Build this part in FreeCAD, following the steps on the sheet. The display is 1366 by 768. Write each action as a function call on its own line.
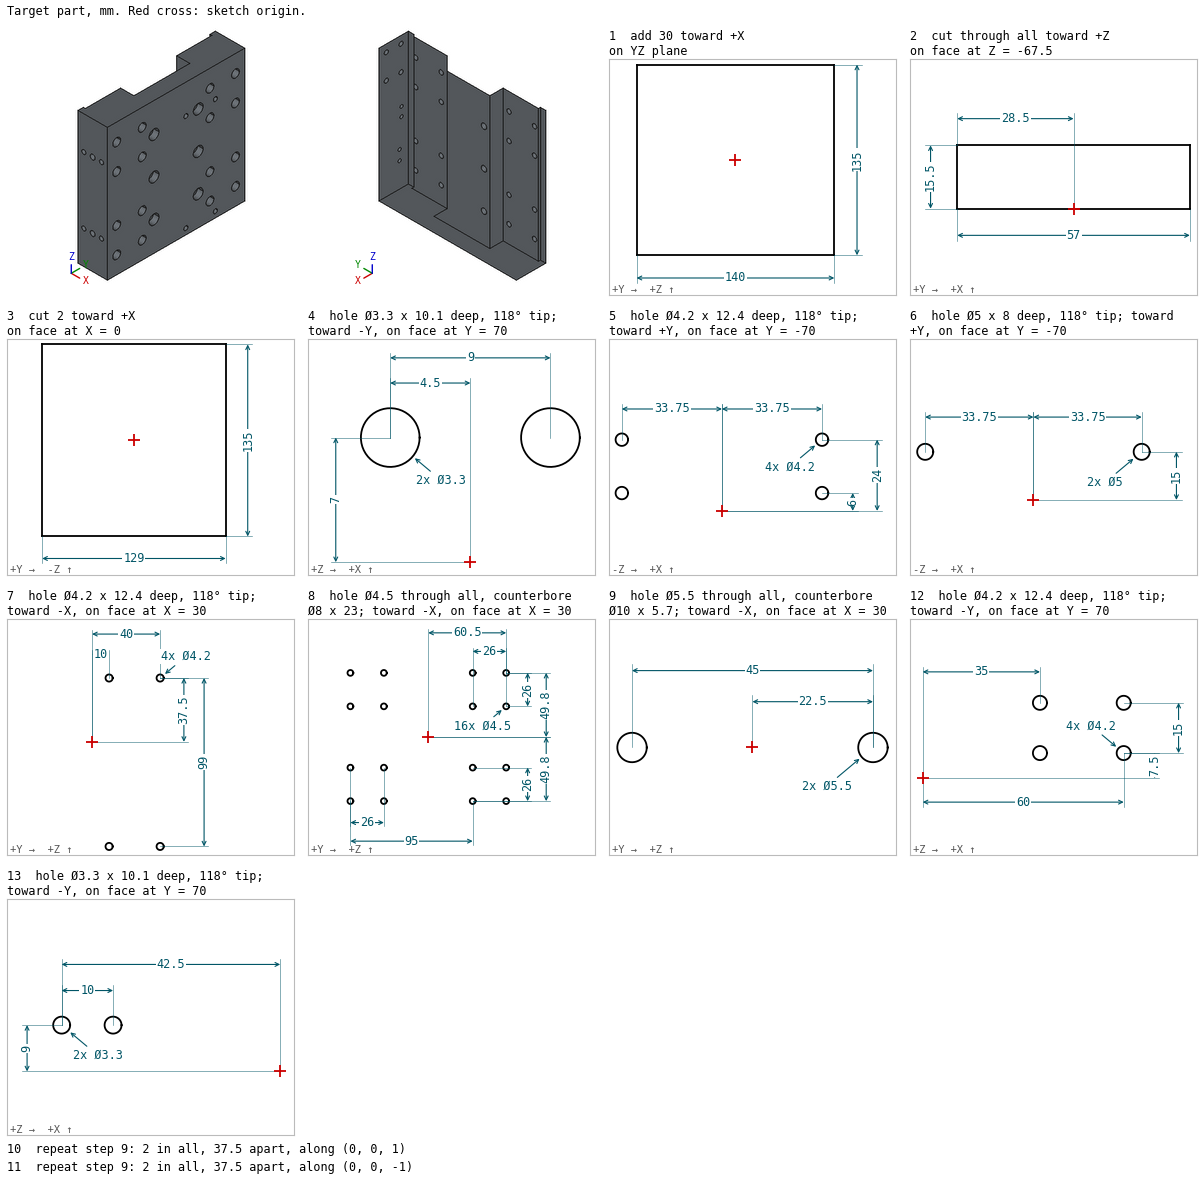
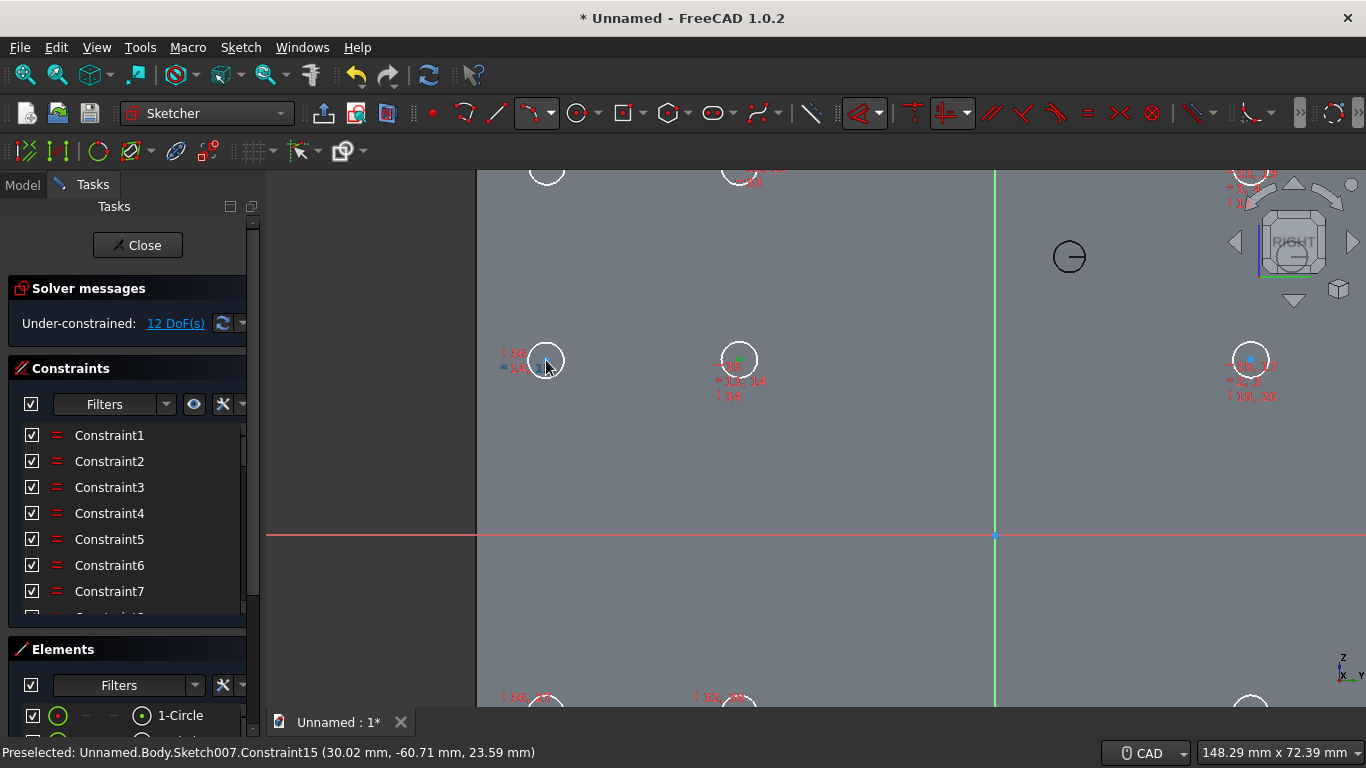
click(546, 361)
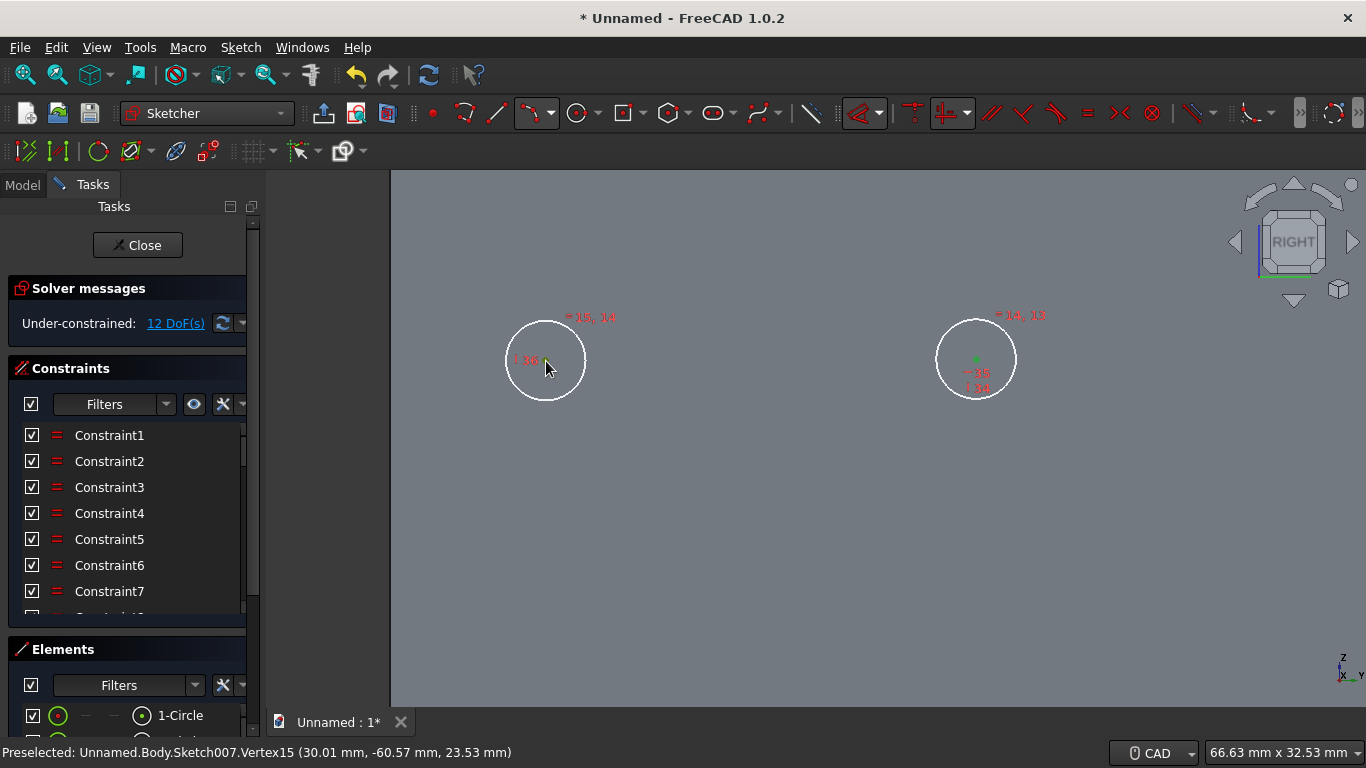
click(970, 114)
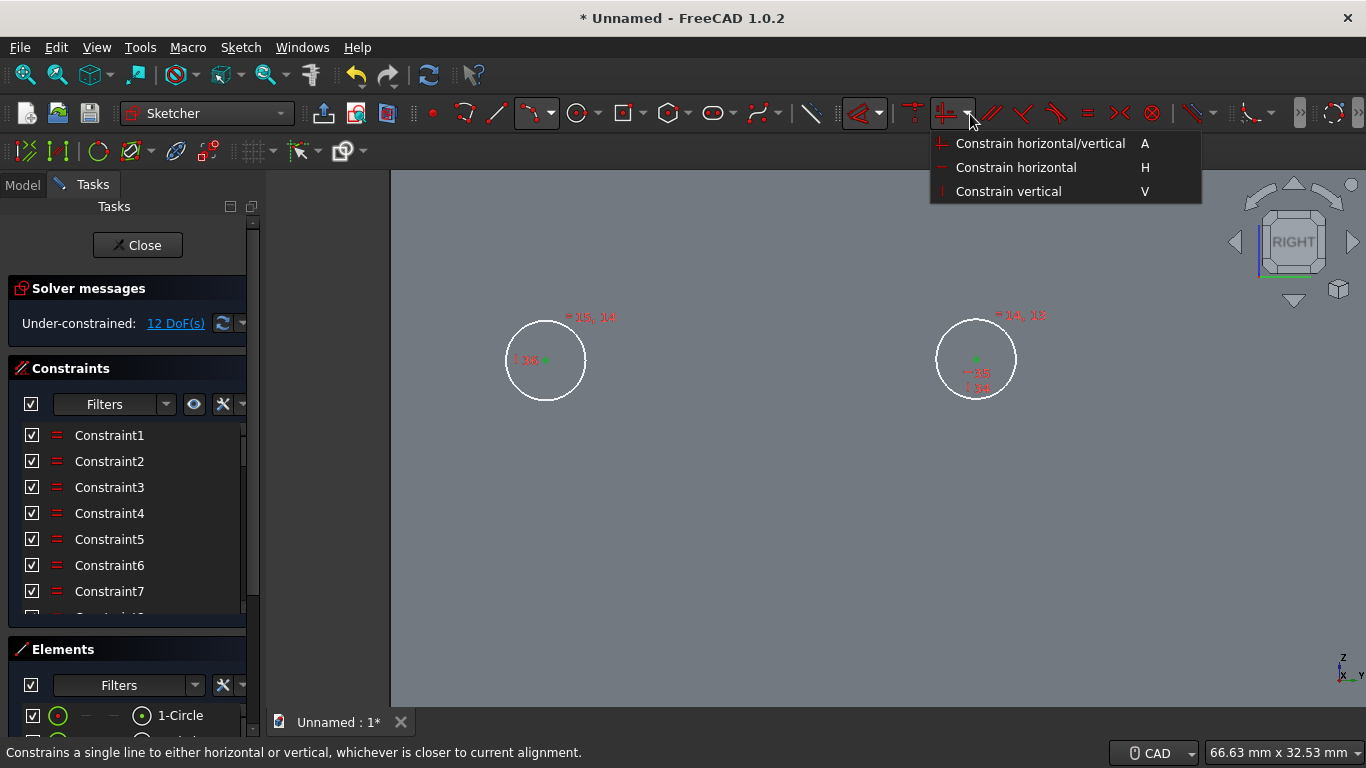
click(1066, 167)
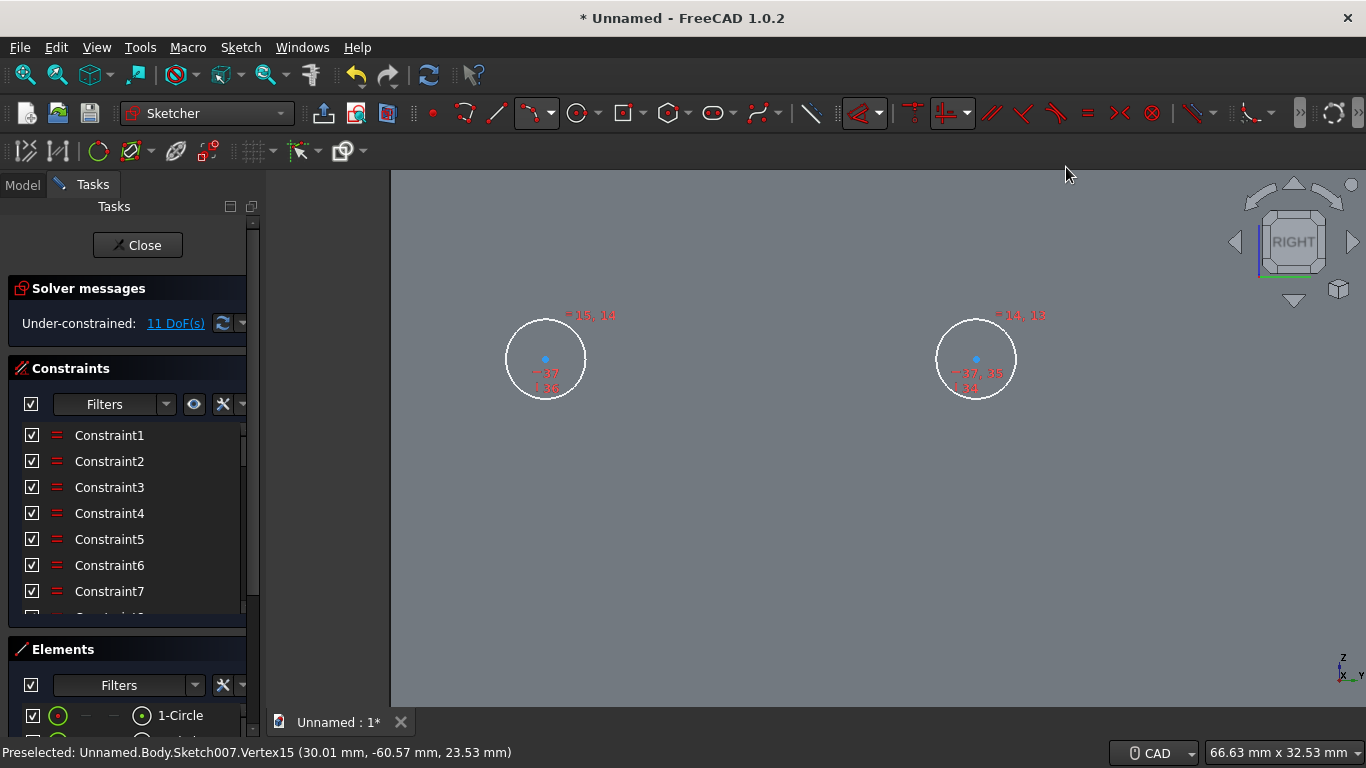
scroll(546, 360, down, 8)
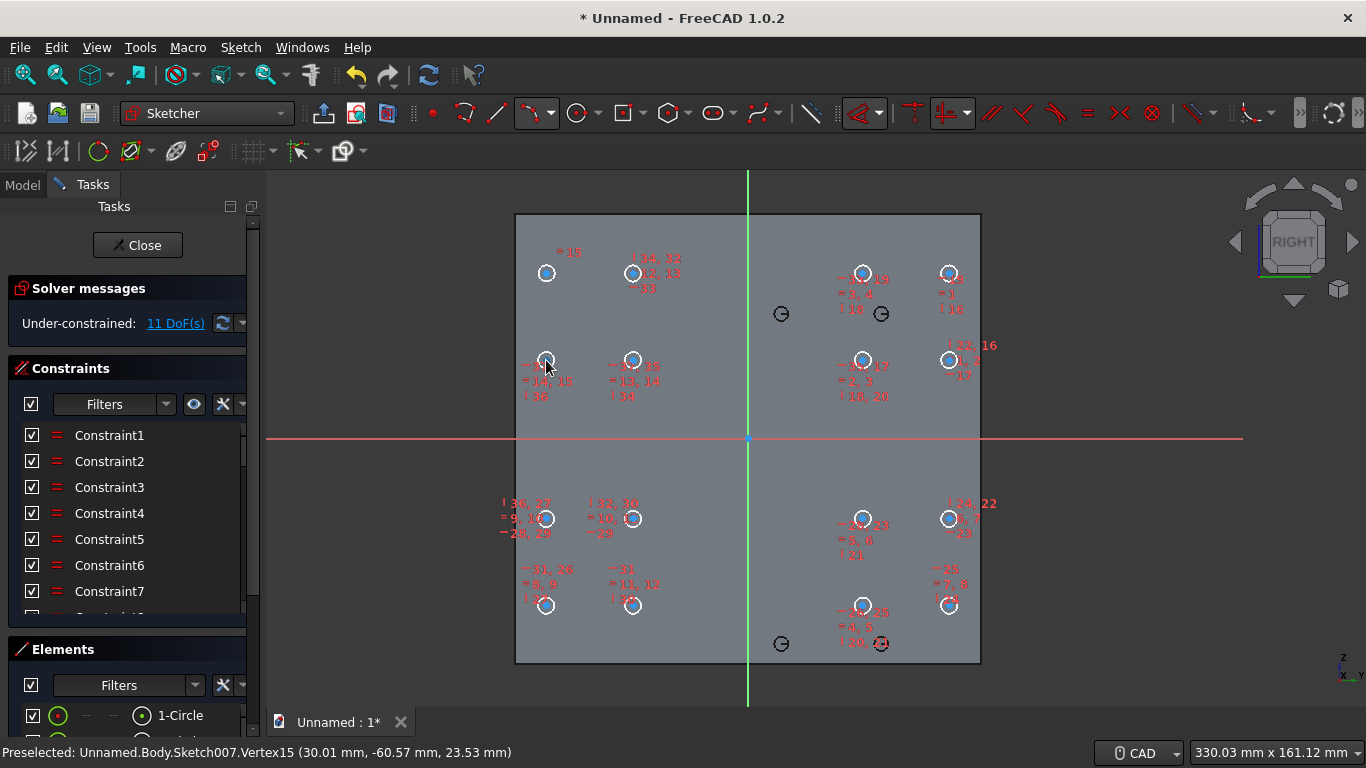
click(544, 358)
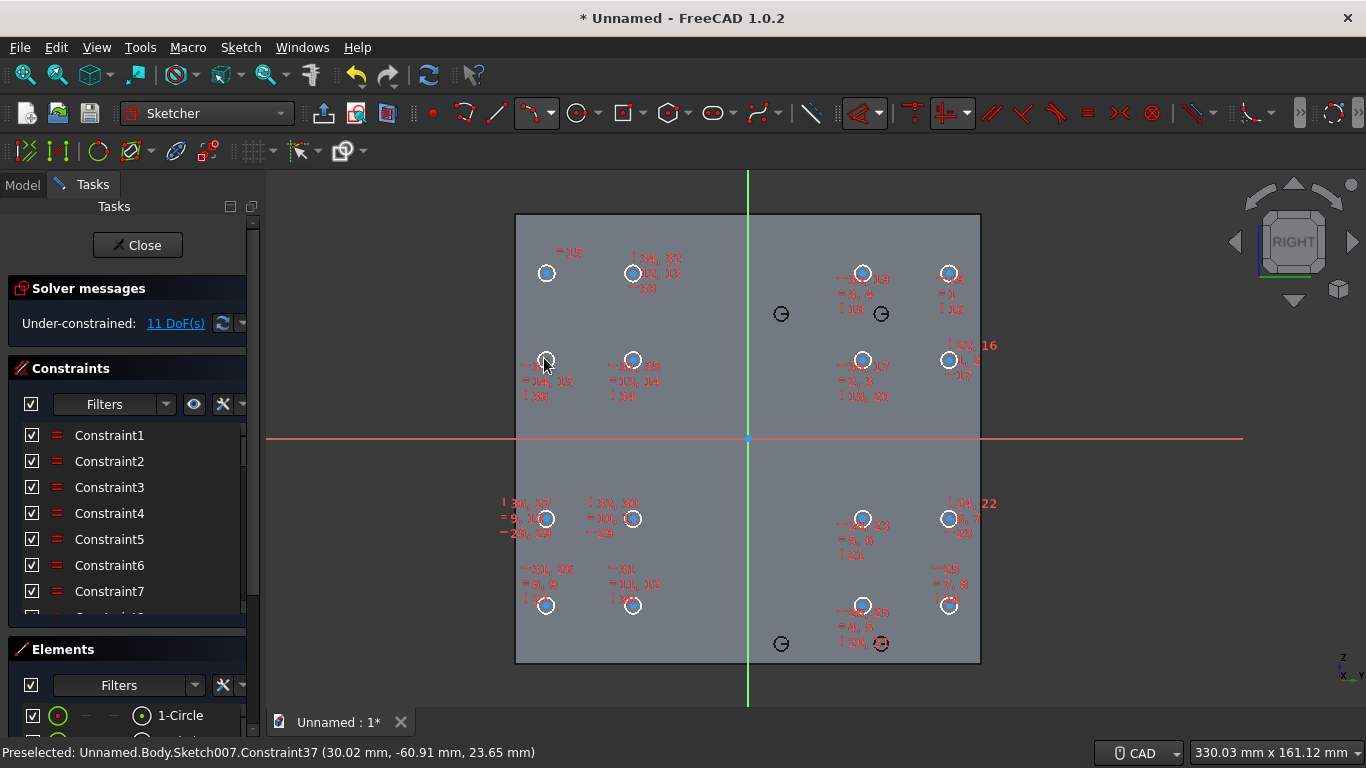
click(547, 273)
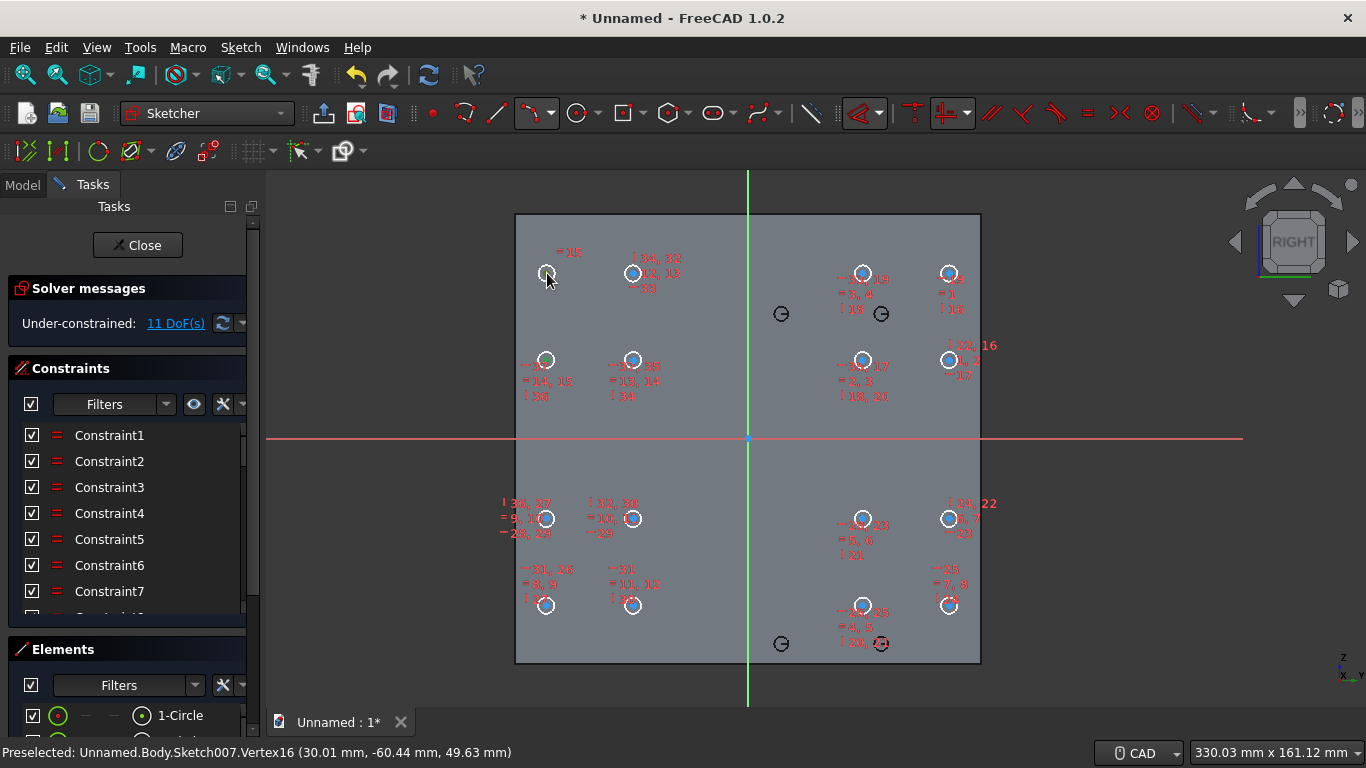
key(v)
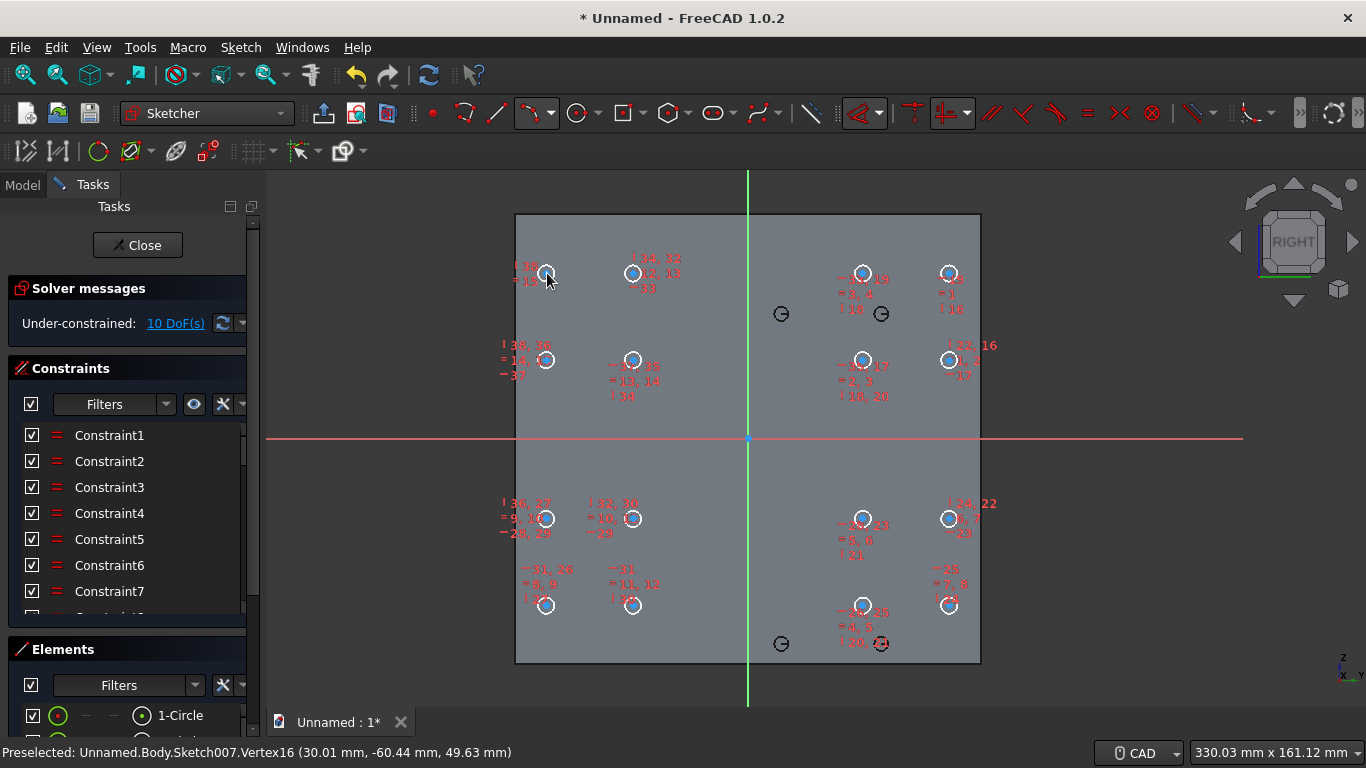
click(633, 273)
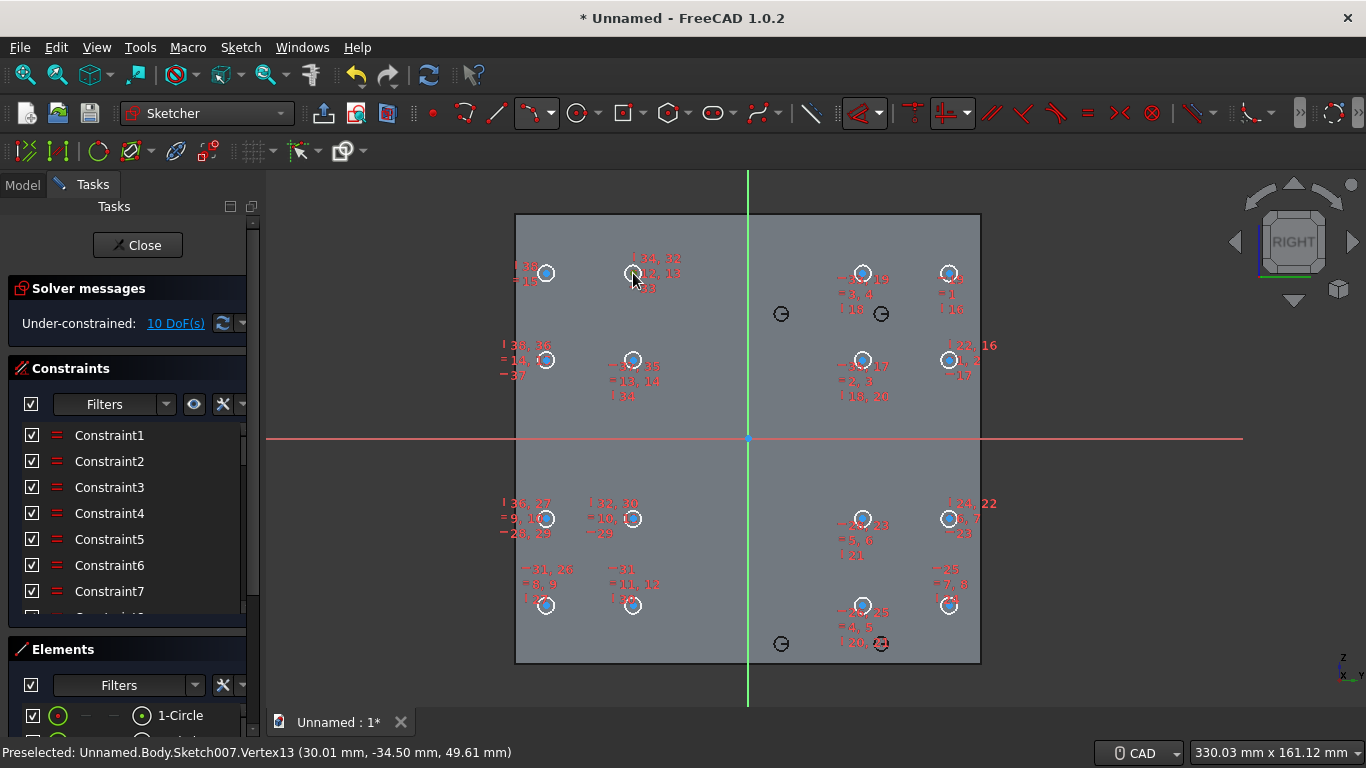
click(546, 273)